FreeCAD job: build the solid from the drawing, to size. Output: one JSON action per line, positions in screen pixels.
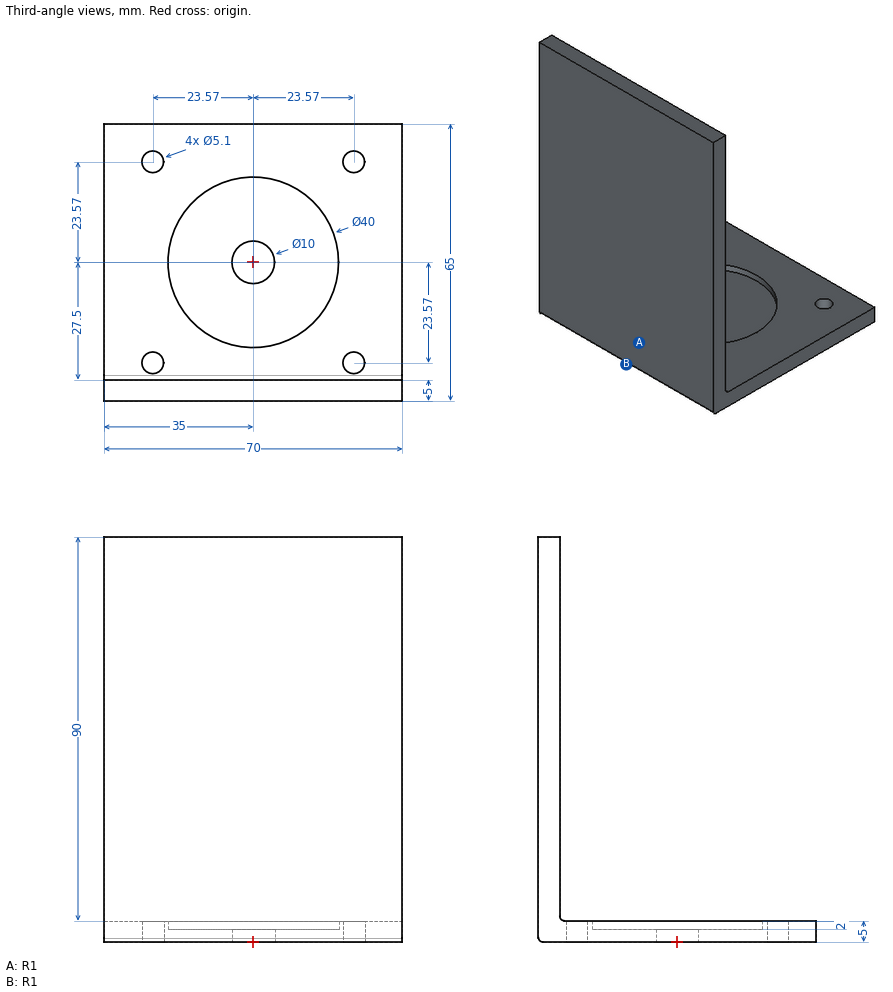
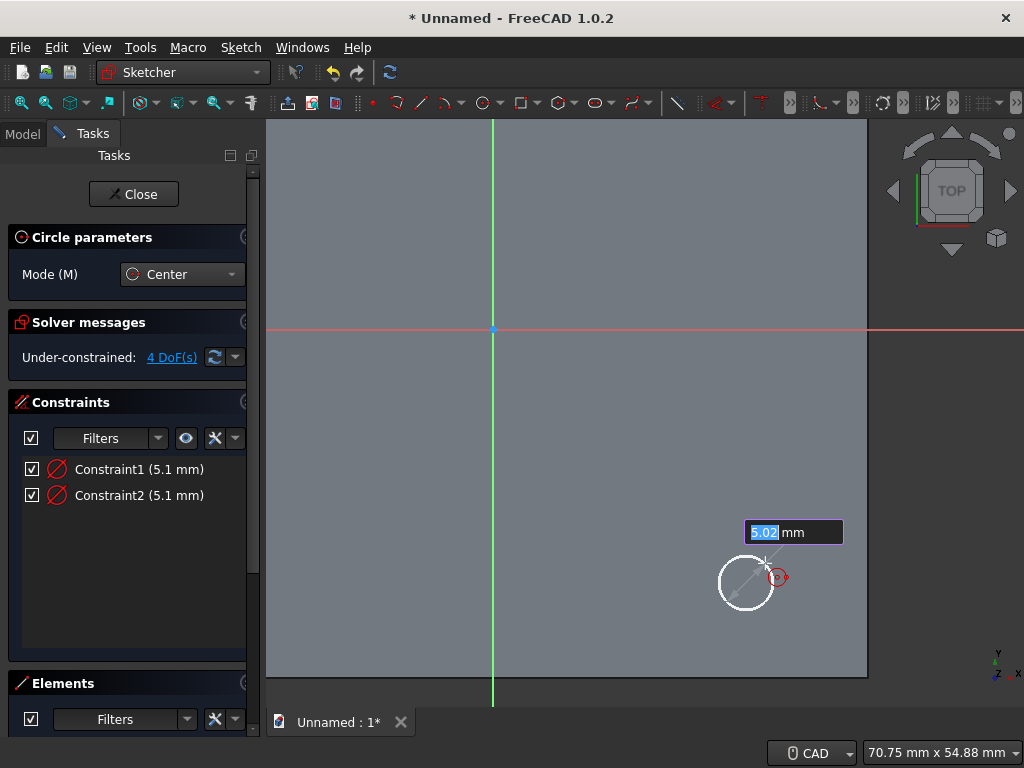
{"action": "type", "text": "5.1"}
{"action": "key", "text": "Return"}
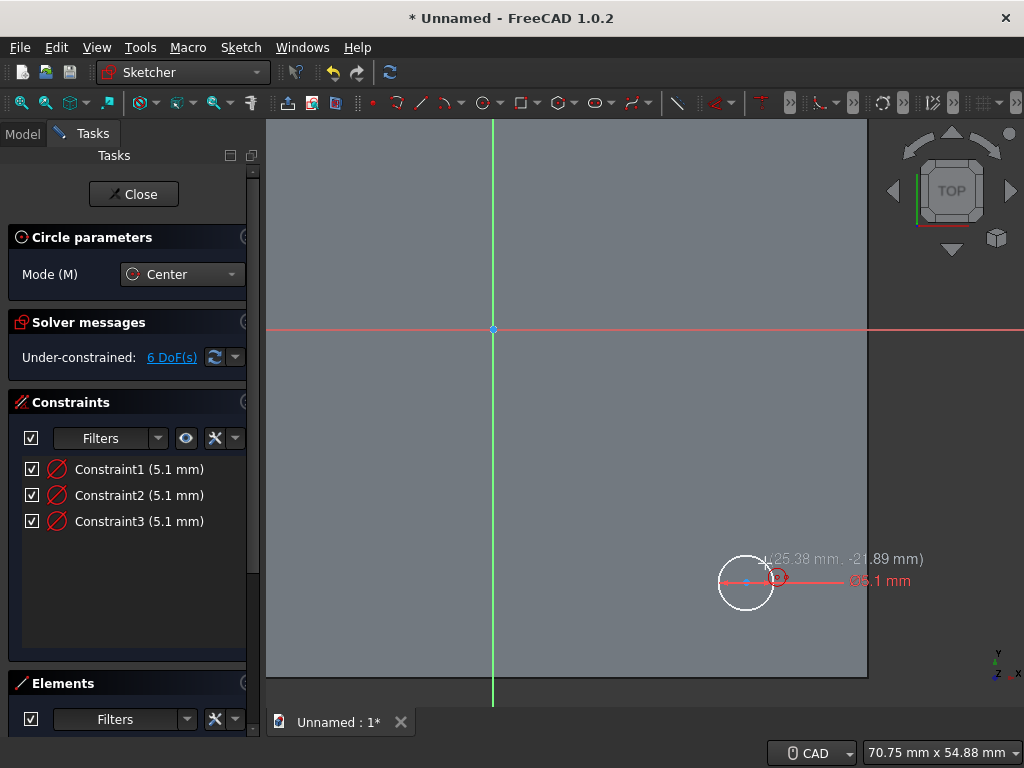
{"action": "scroll", "coordinate": [746, 583], "scroll_direction": "down", "scroll_amount": 2}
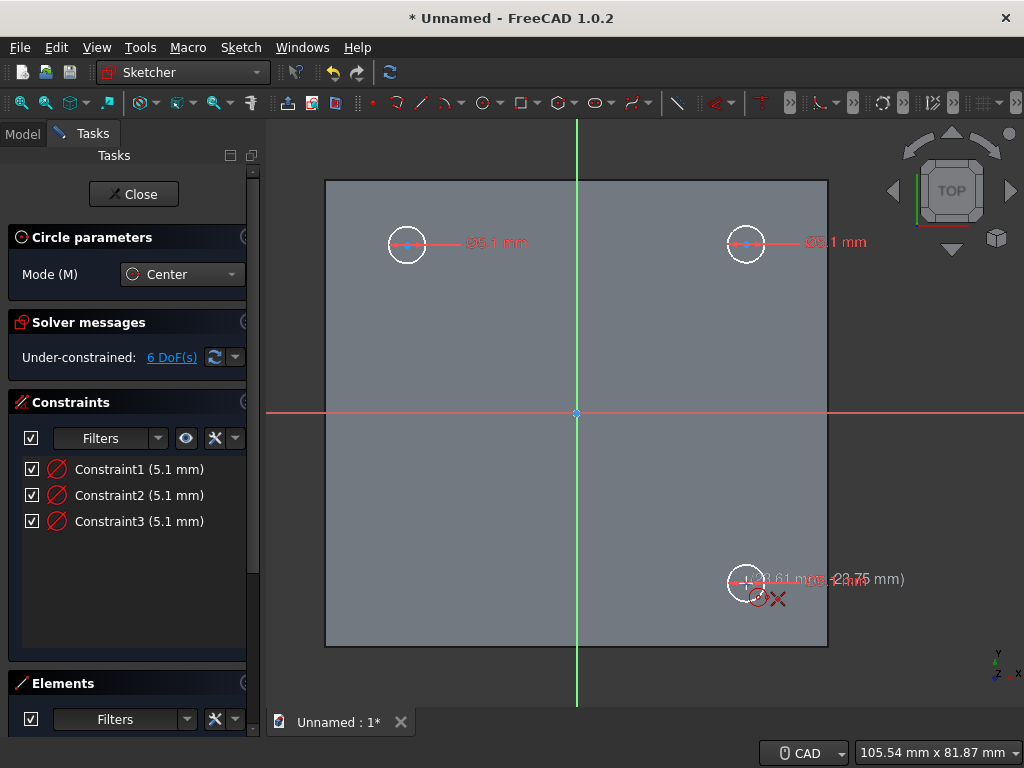
{"action": "scroll", "coordinate": [407, 583], "scroll_direction": "up", "scroll_amount": 2}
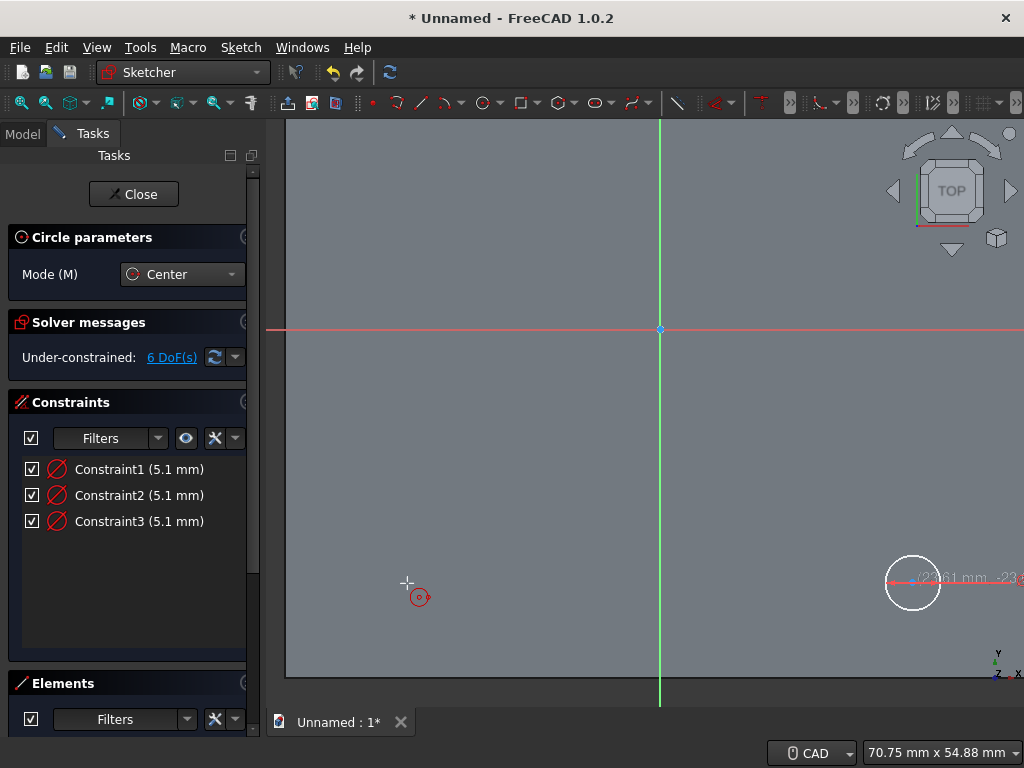
{"action": "left_click", "coordinate": [407, 582]}
{"action": "mouse_move", "coordinate": [427, 563]}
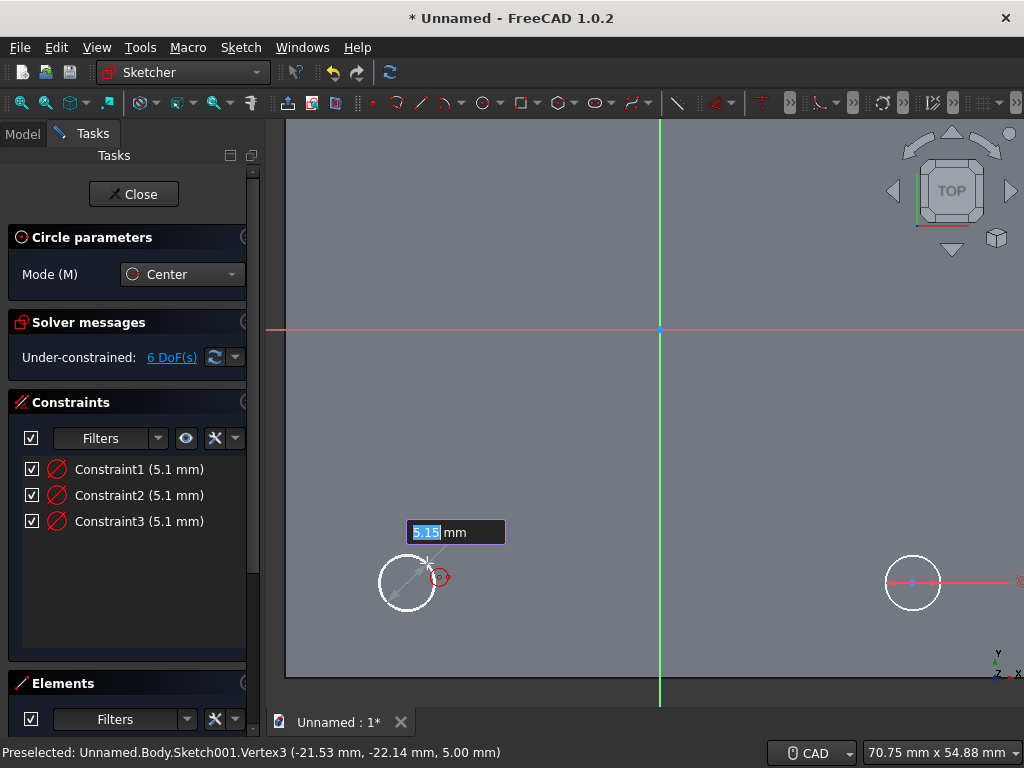
{"action": "type", "text": "5.1"}
{"action": "key", "text": "Return"}
{"action": "key", "text": "Escape"}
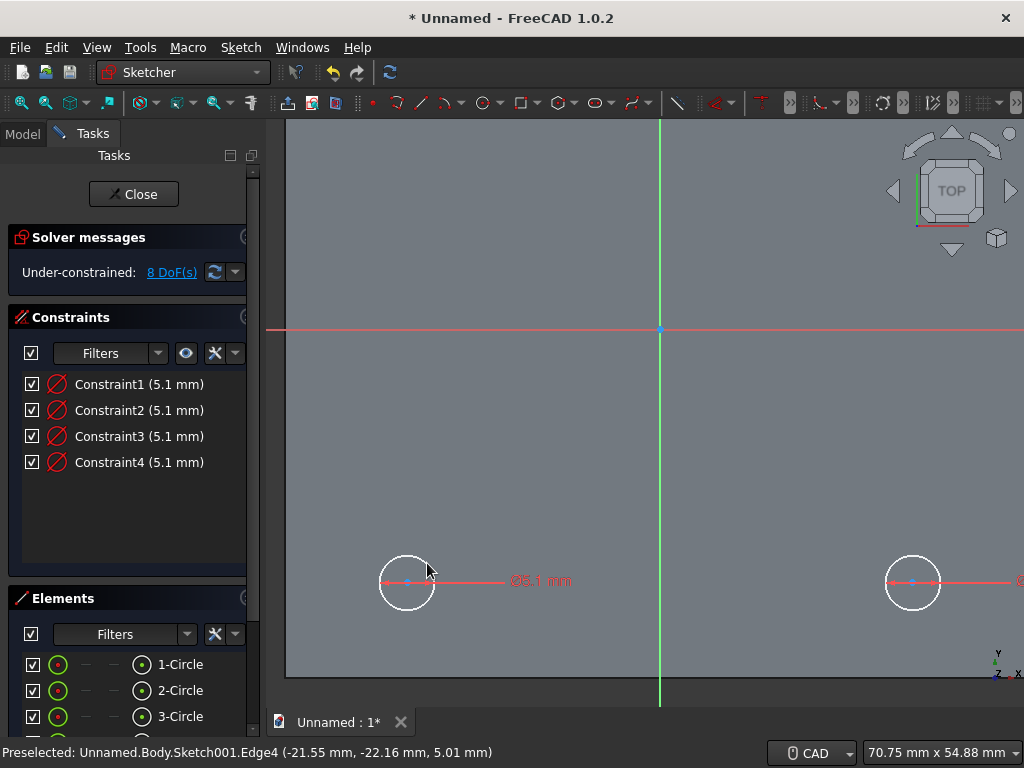
{"action": "scroll", "coordinate": [407, 583], "scroll_direction": "down", "scroll_amount": 2}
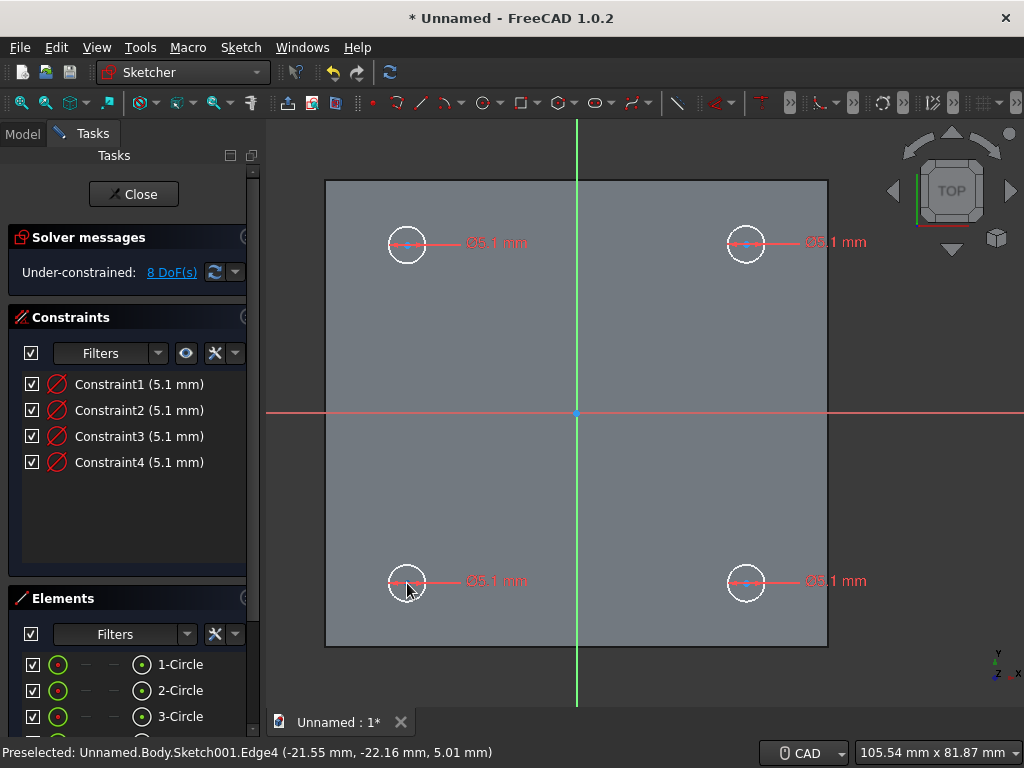
{"action": "left_click", "coordinate": [407, 245]}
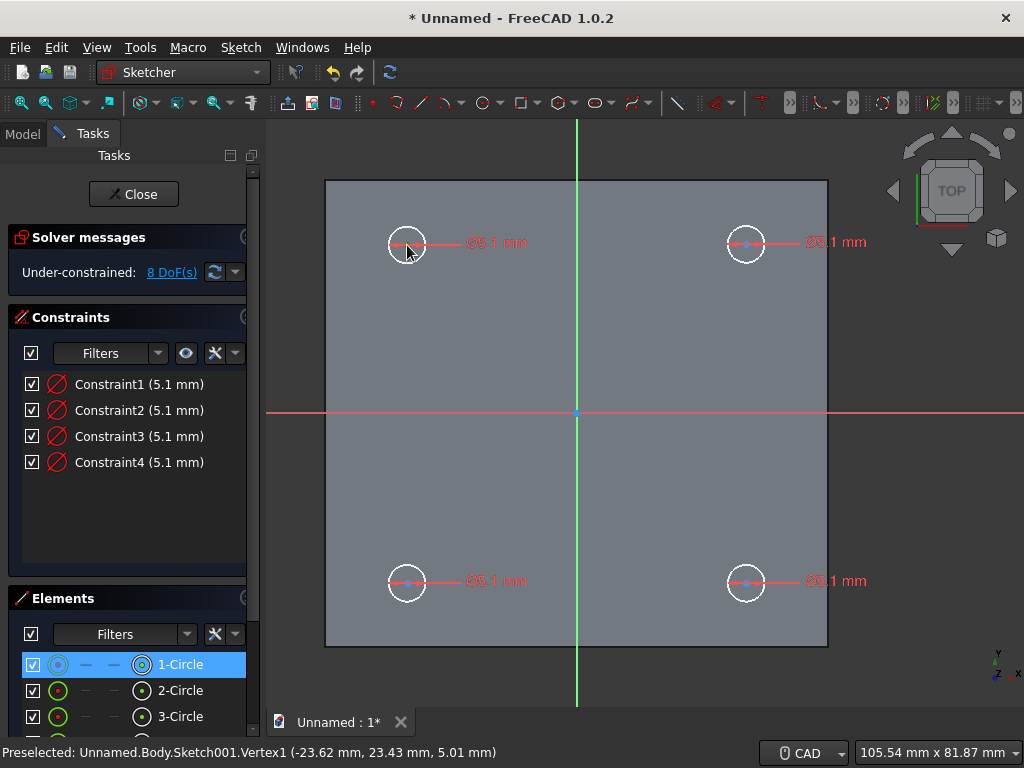
{"action": "left_click", "coordinate": [746, 244]}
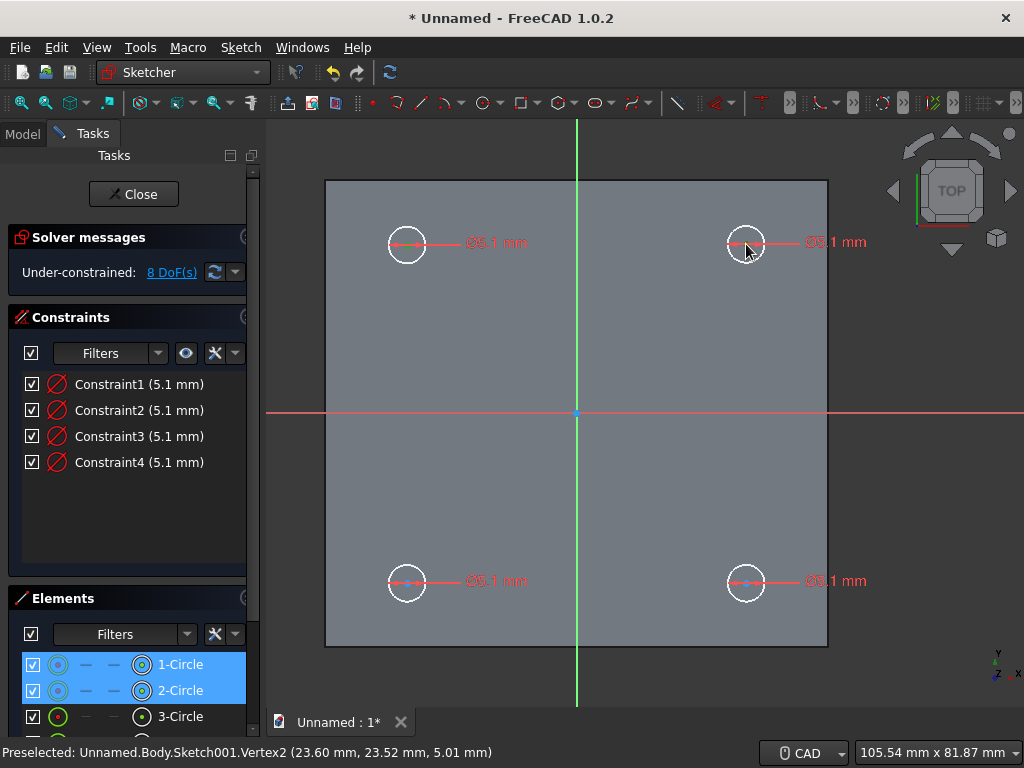
{"action": "key", "text": "h"}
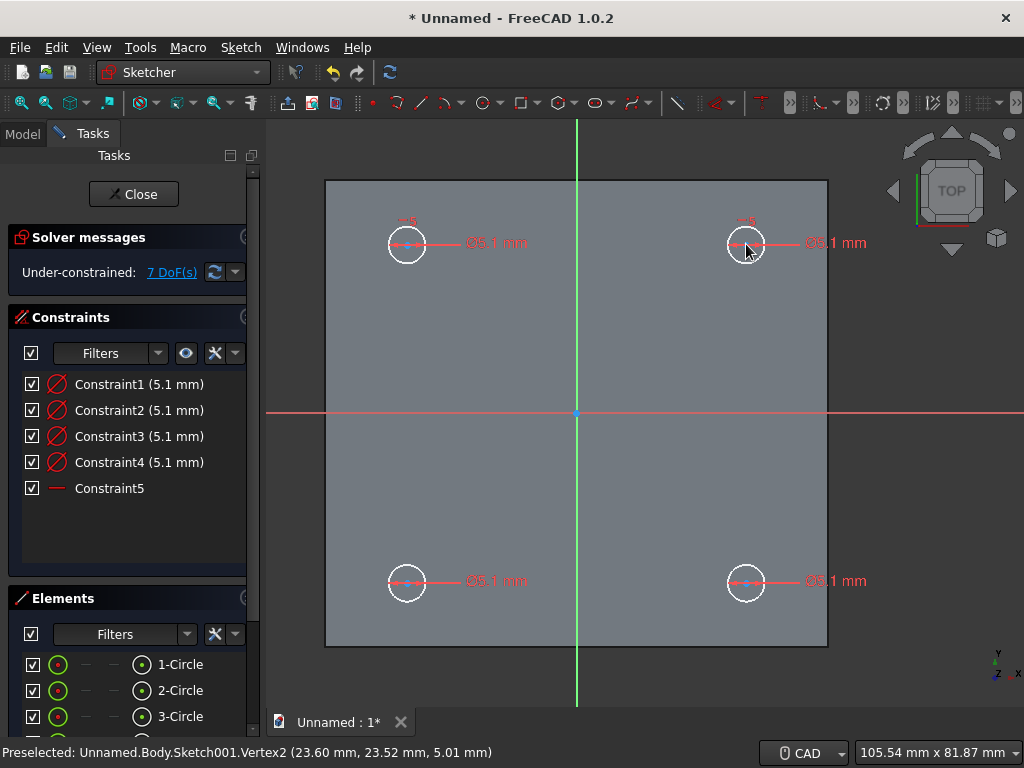
{"action": "left_click", "coordinate": [746, 245]}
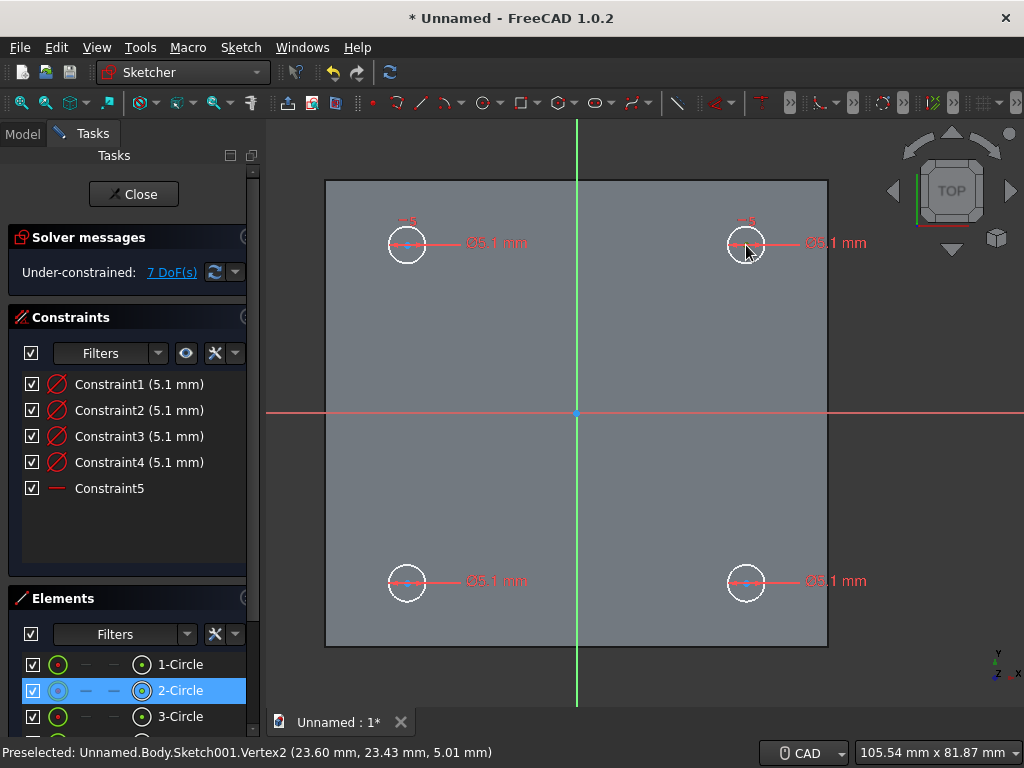
{"action": "left_click", "coordinate": [746, 583]}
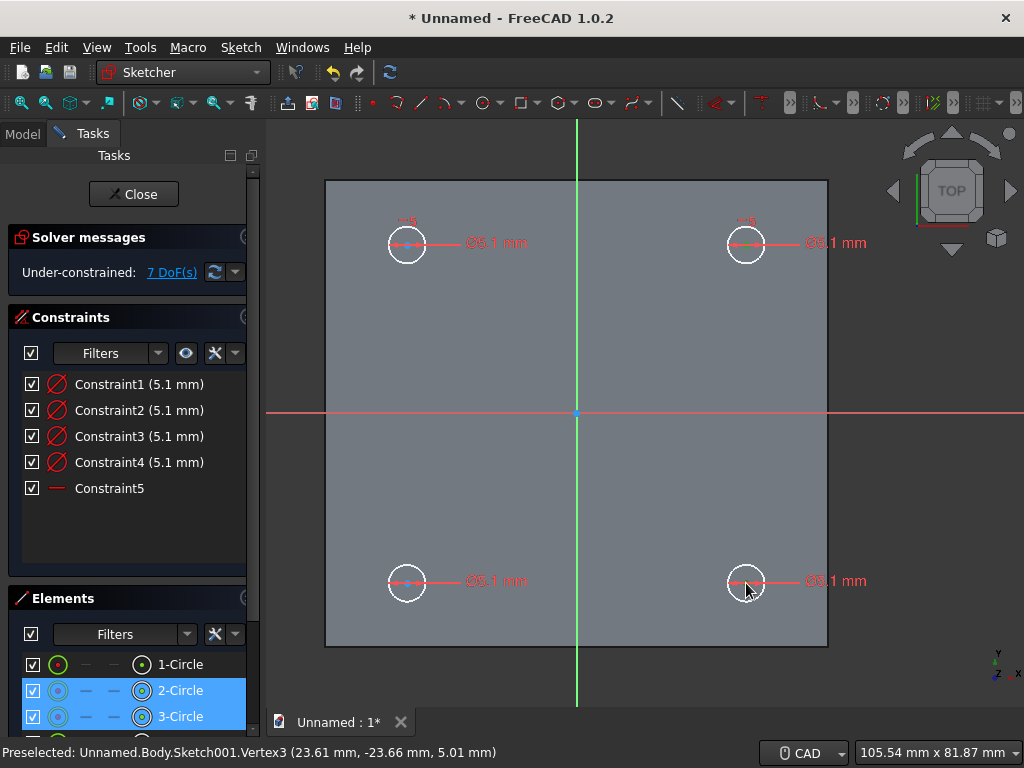
{"action": "key", "text": "v"}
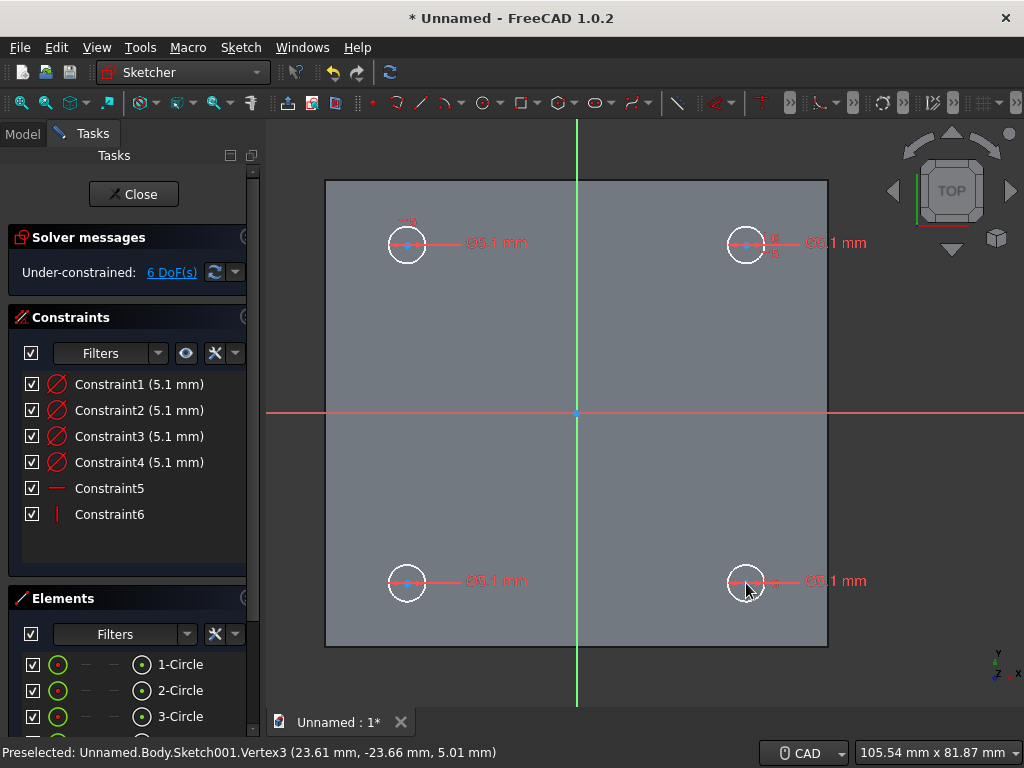
{"action": "left_click", "coordinate": [407, 245]}